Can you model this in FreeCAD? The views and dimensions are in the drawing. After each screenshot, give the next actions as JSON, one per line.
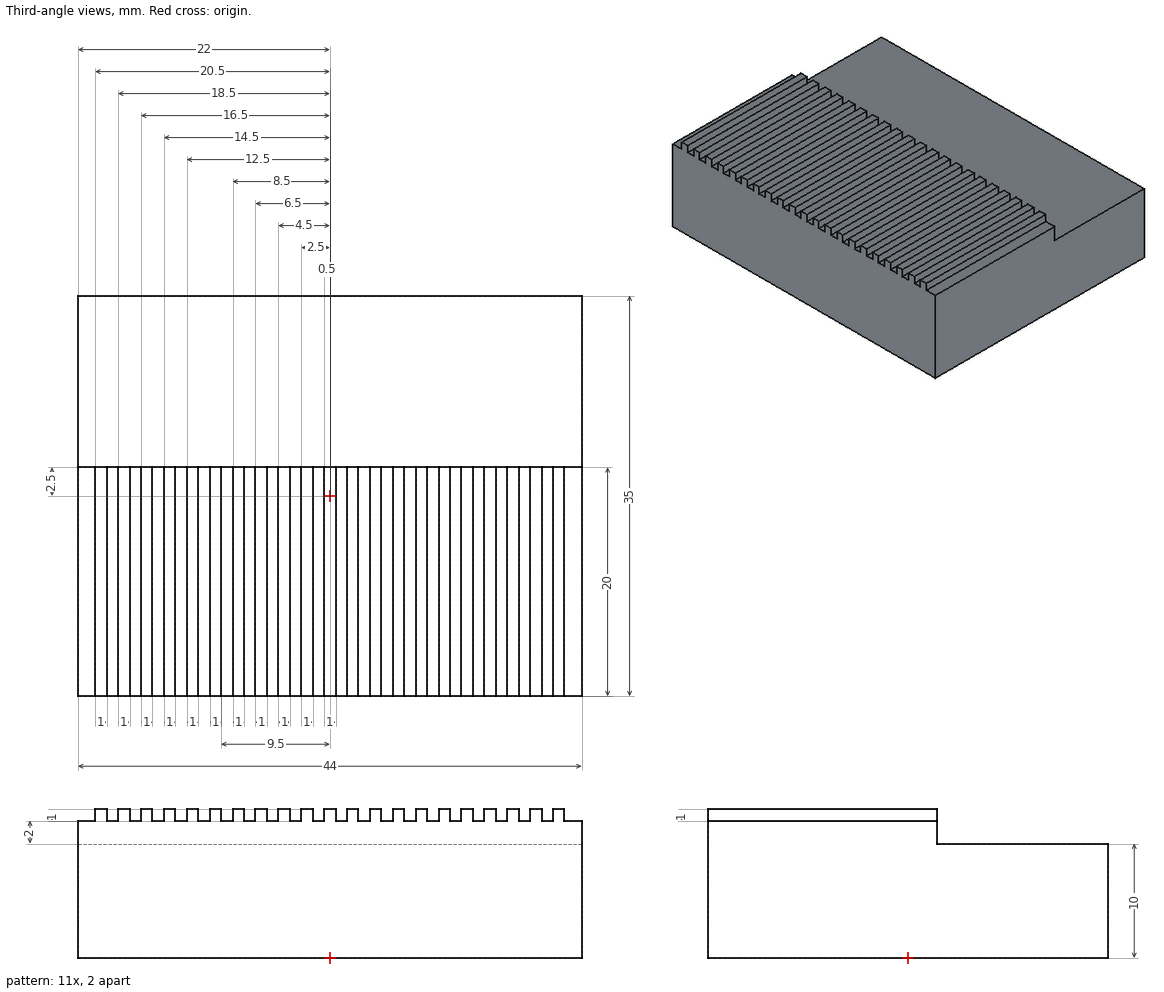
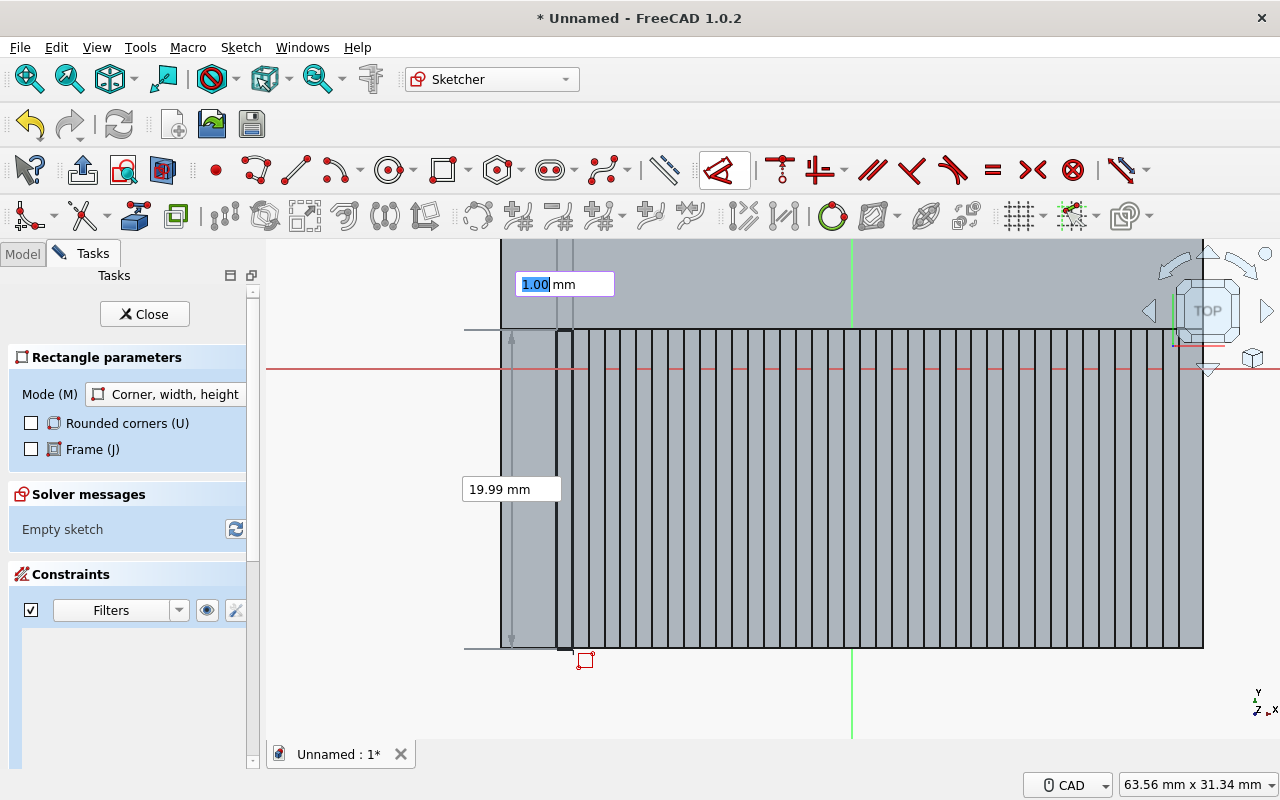
{"action": "type", "text": "1"}
{"action": "key", "text": "Tab"}
{"action": "type", "text": "20"}
{"action": "key", "text": "Return"}
{"action": "key", "text": "Escape"}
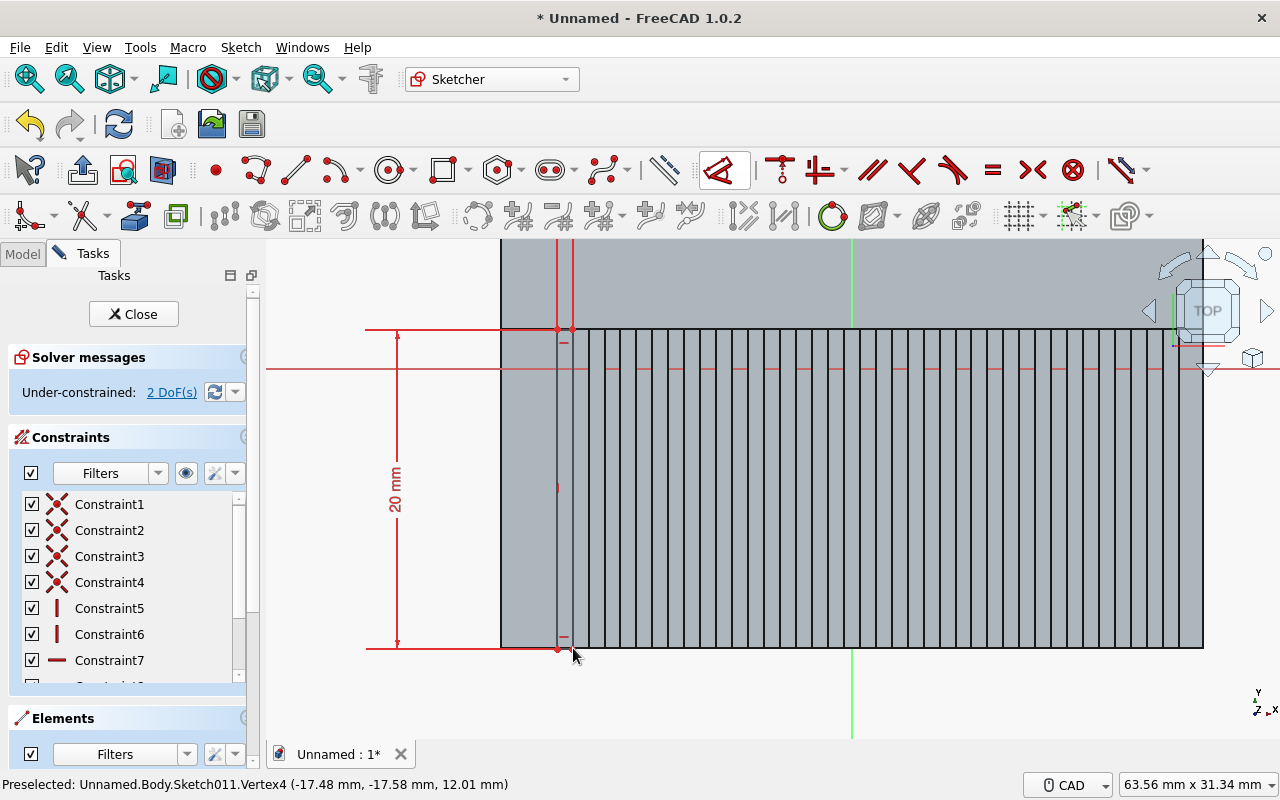
{"action": "left_click", "coordinate": [557, 330]}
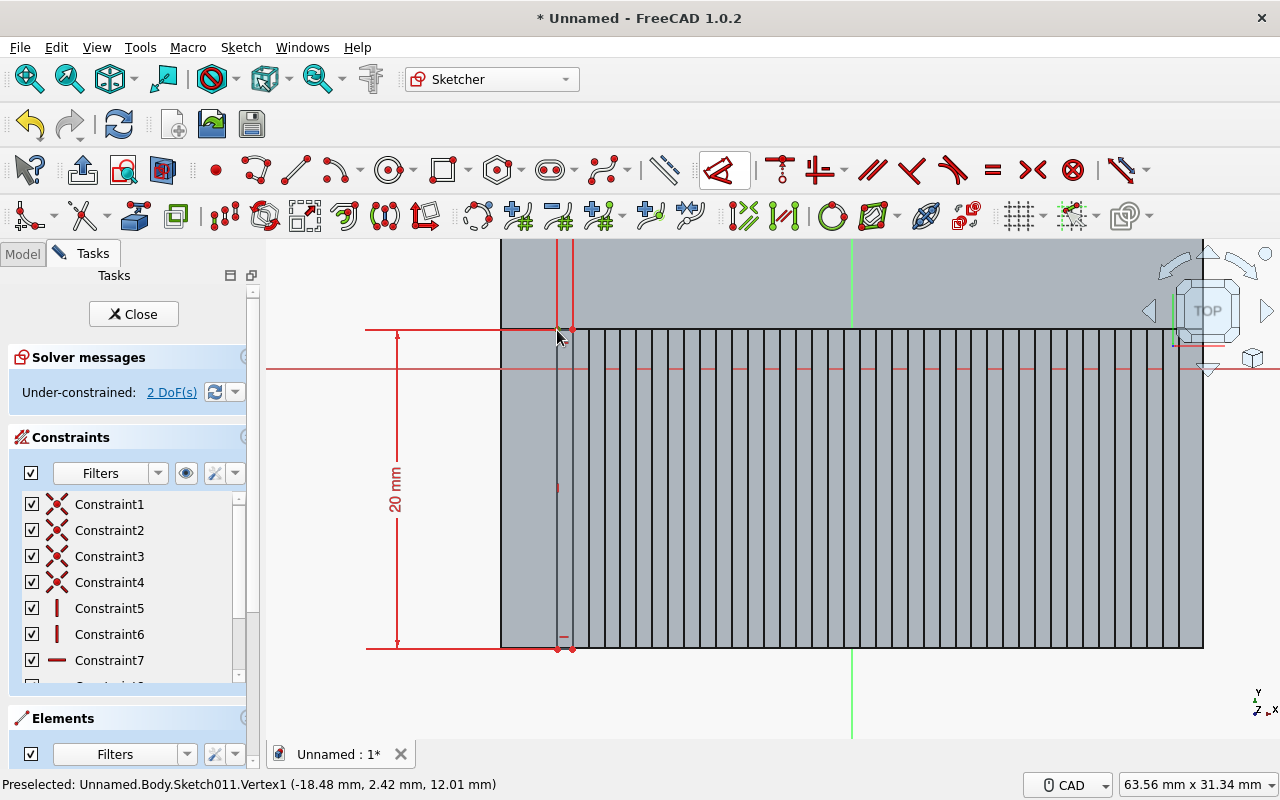
{"action": "key", "text": "i"}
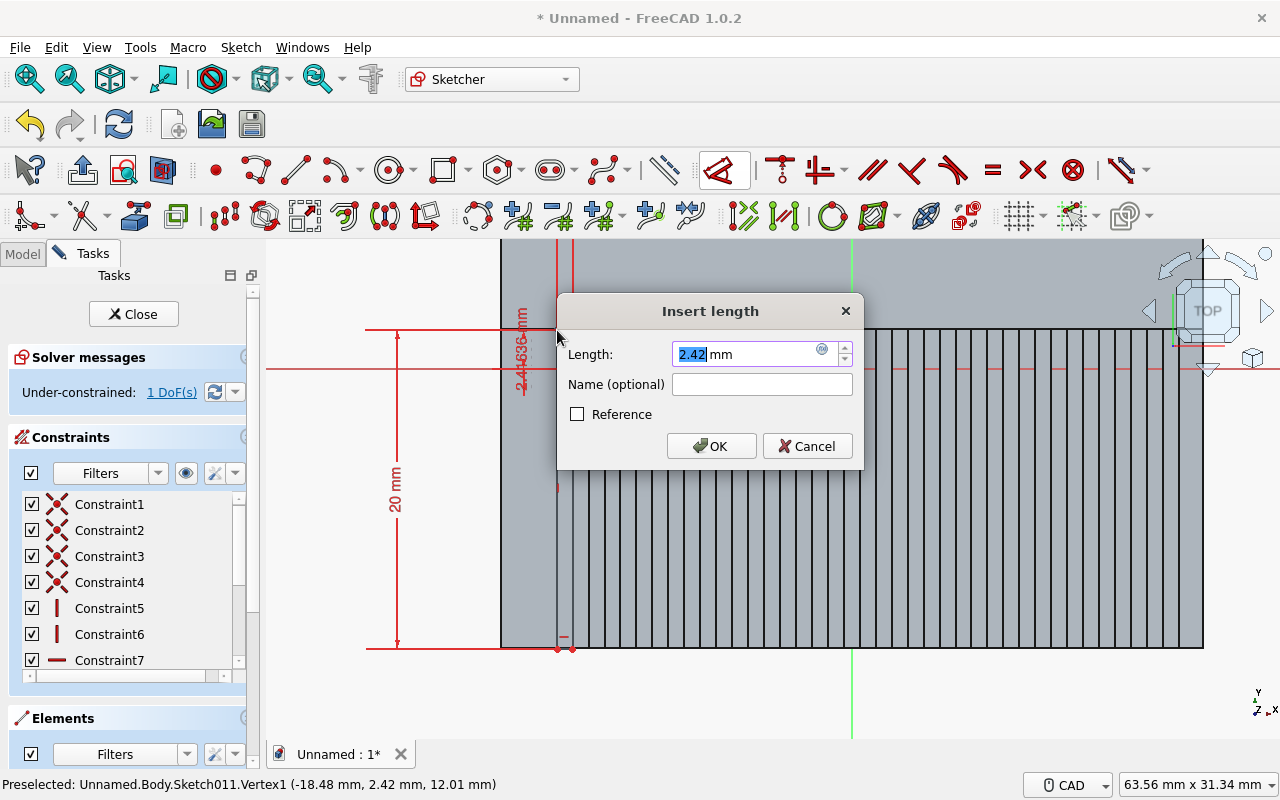
{"action": "type", "text": "2.5"}
{"action": "key", "text": "Return"}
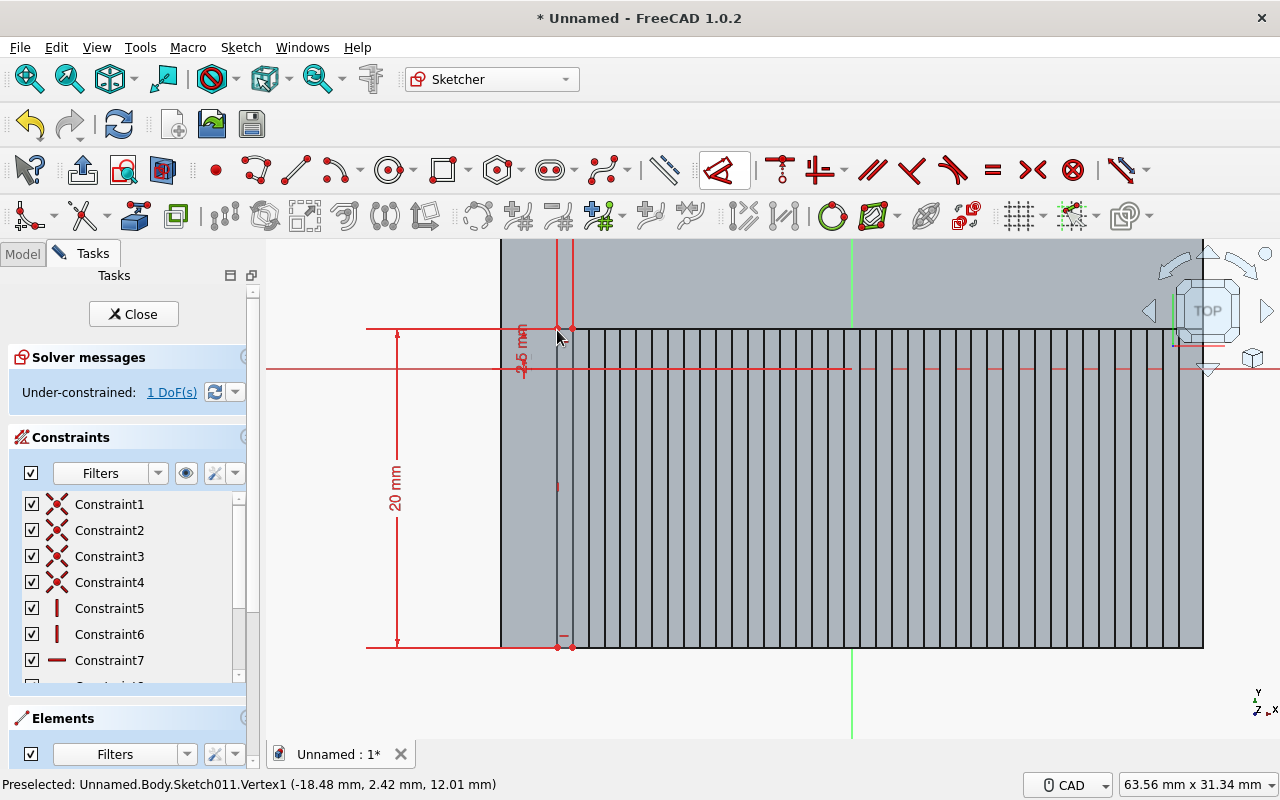
{"action": "left_click", "coordinate": [557, 329]}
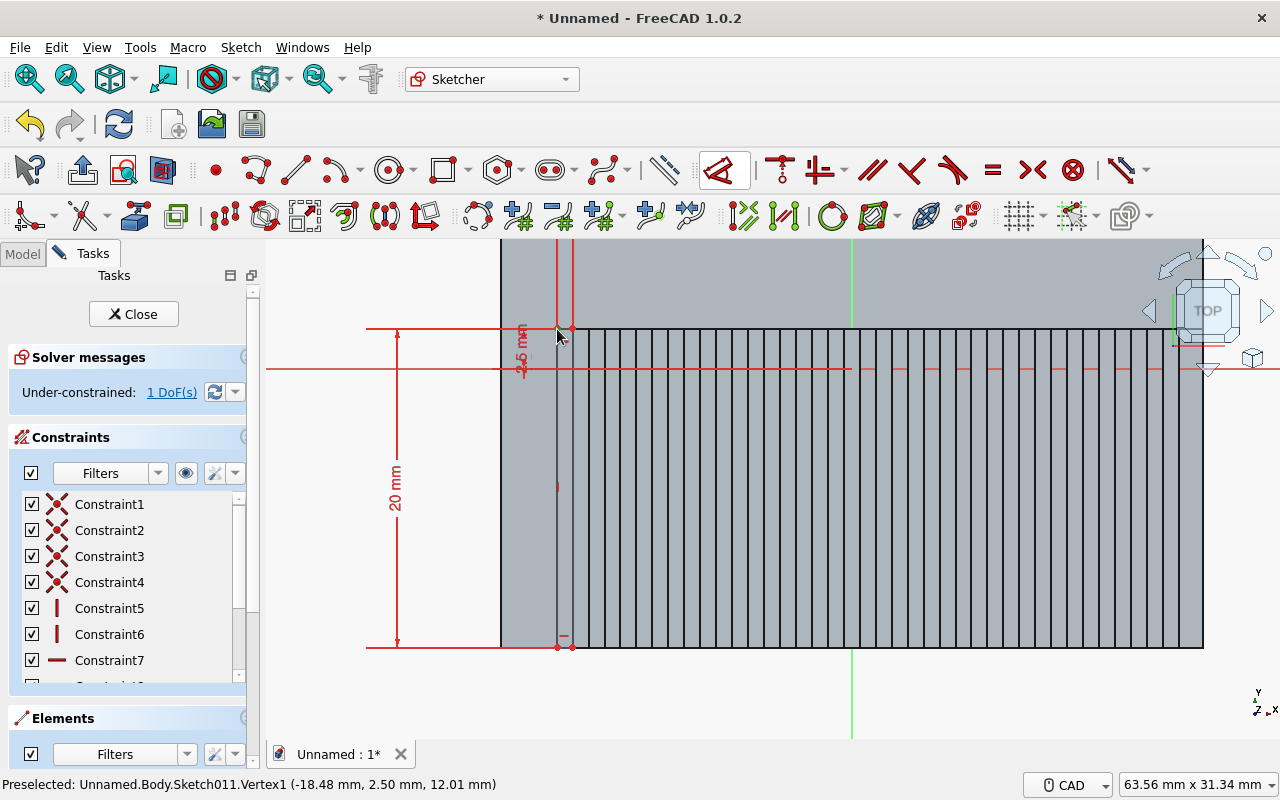
{"action": "key", "text": "l"}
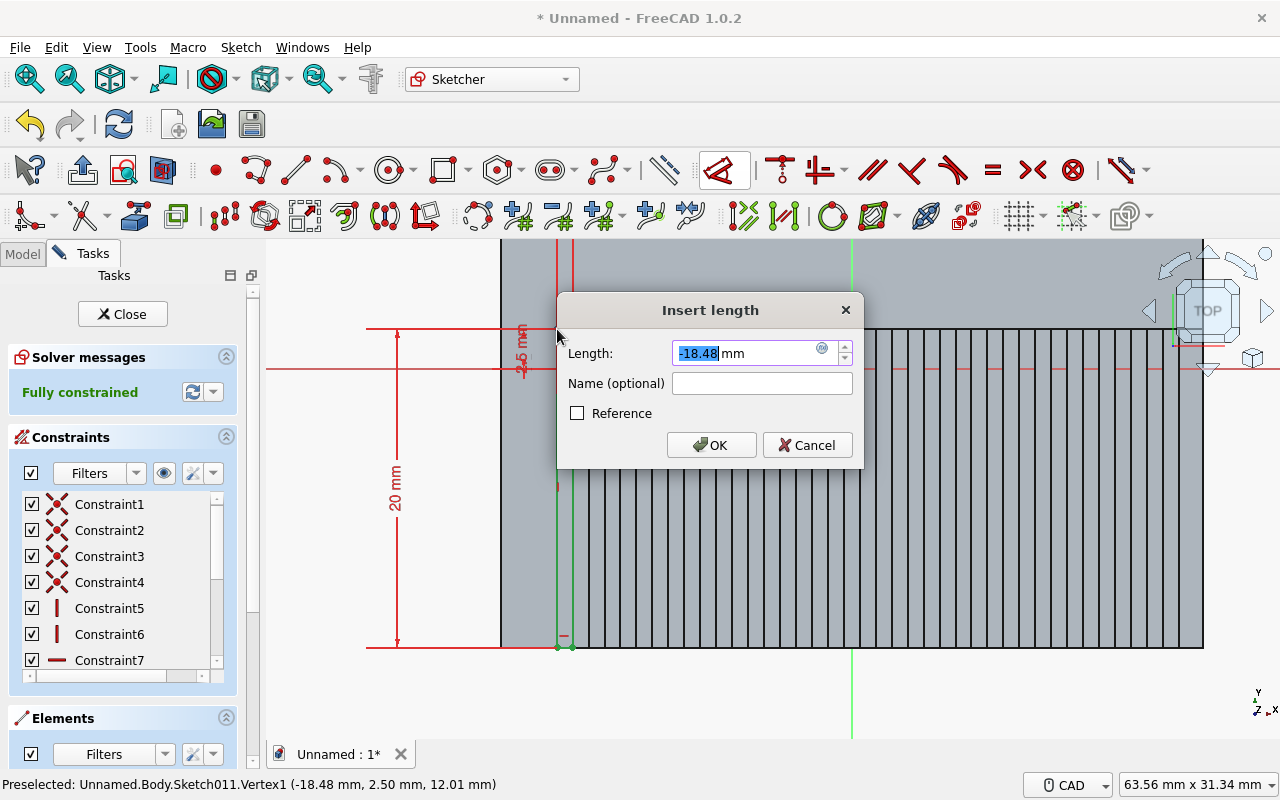
{"action": "type", "text": "-18.5"}
{"action": "key", "text": "Return"}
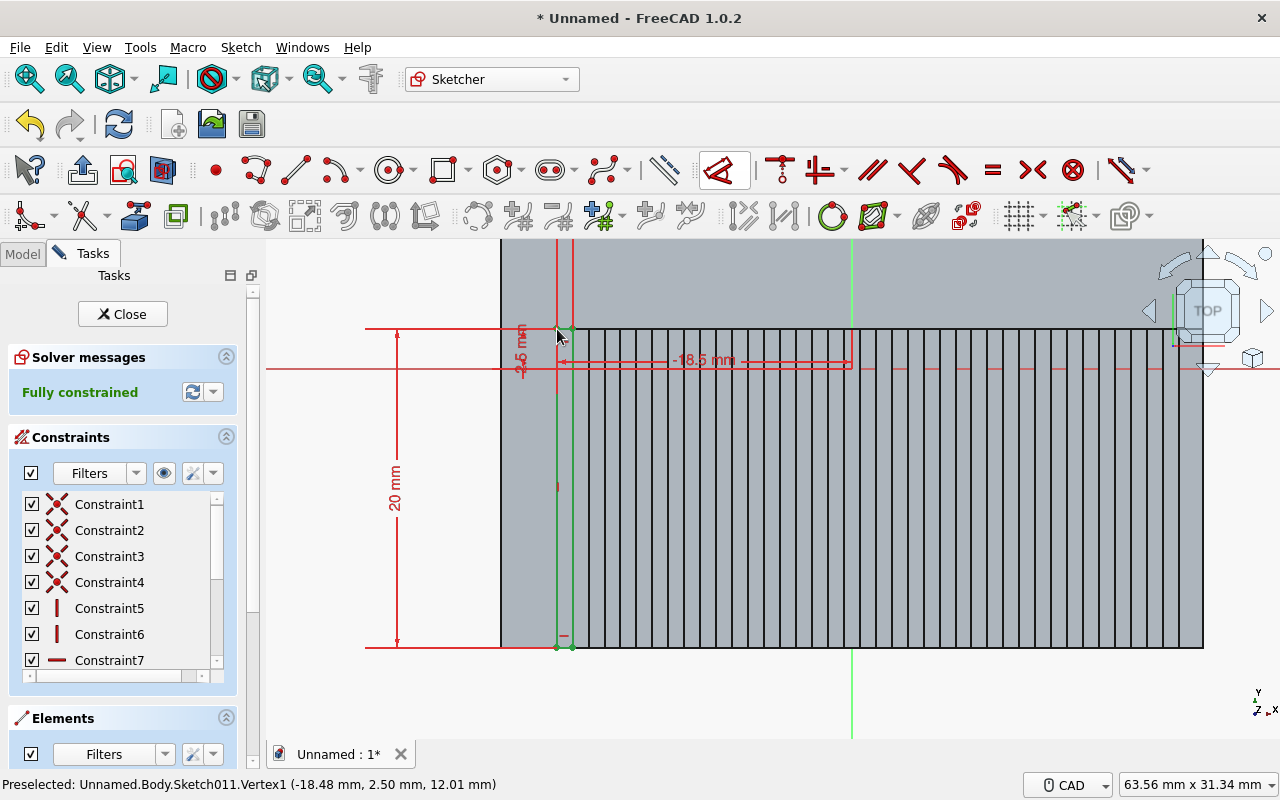
{"action": "left_click", "coordinate": [123, 314]}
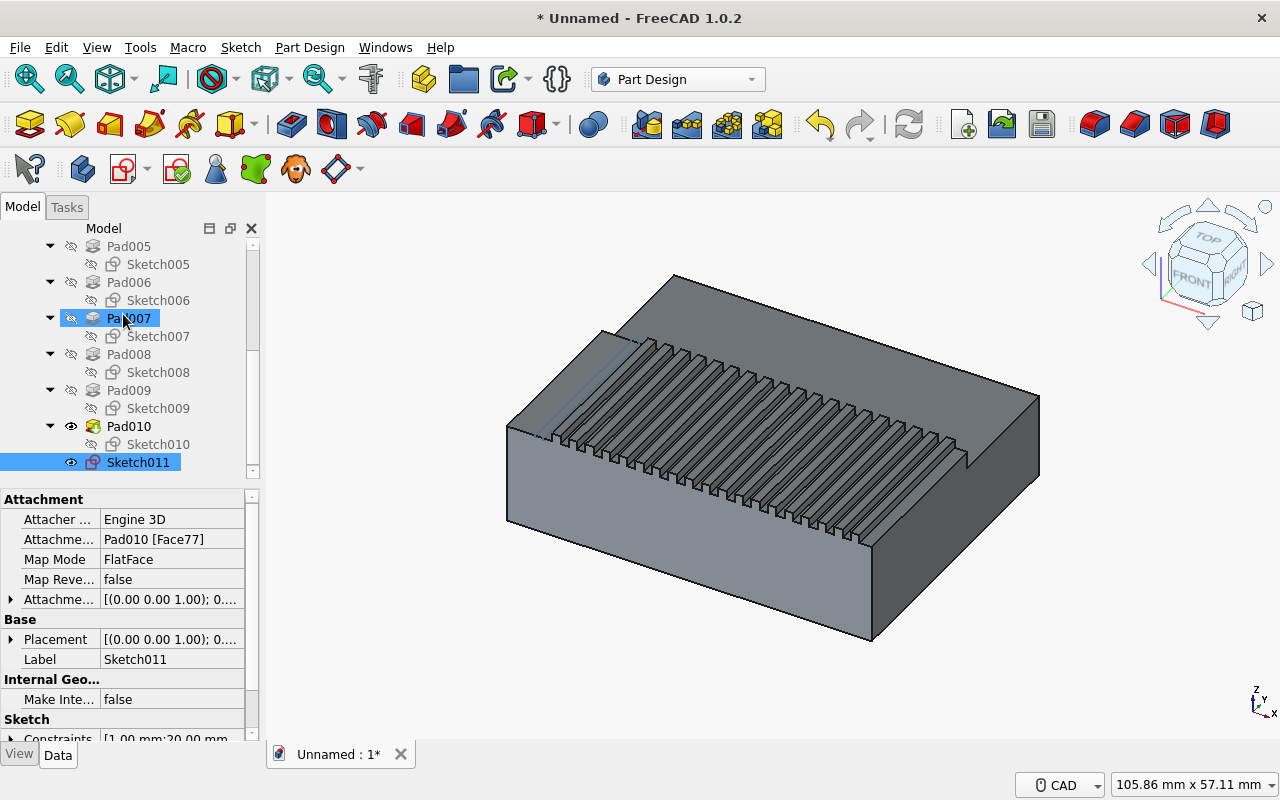
{"action": "left_click", "coordinate": [30, 124]}